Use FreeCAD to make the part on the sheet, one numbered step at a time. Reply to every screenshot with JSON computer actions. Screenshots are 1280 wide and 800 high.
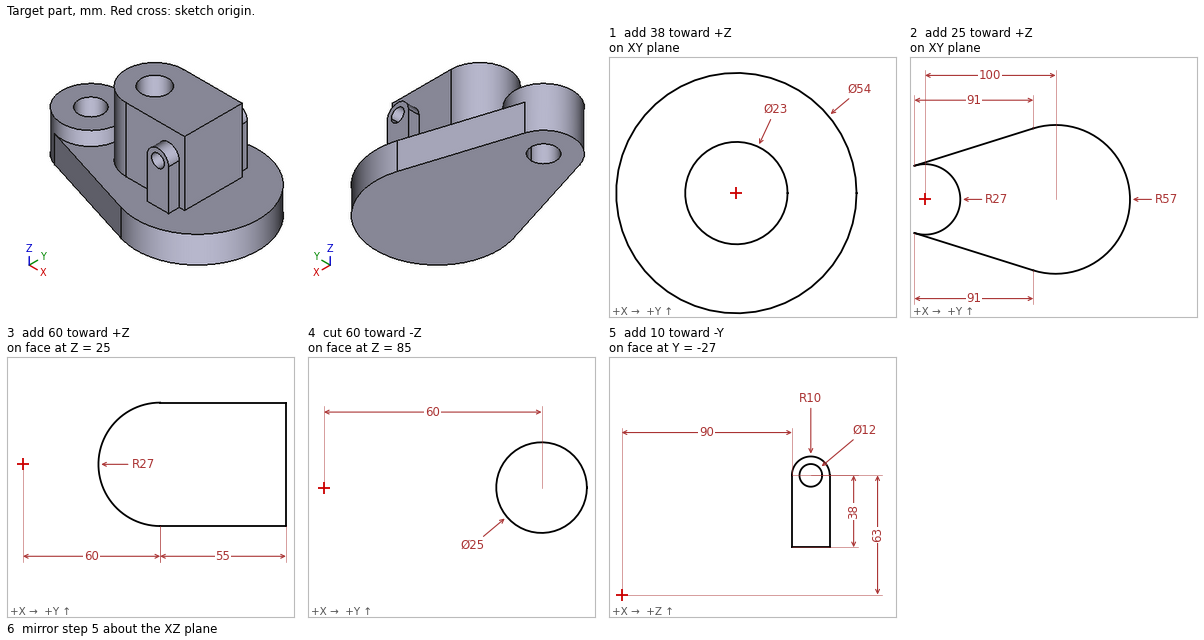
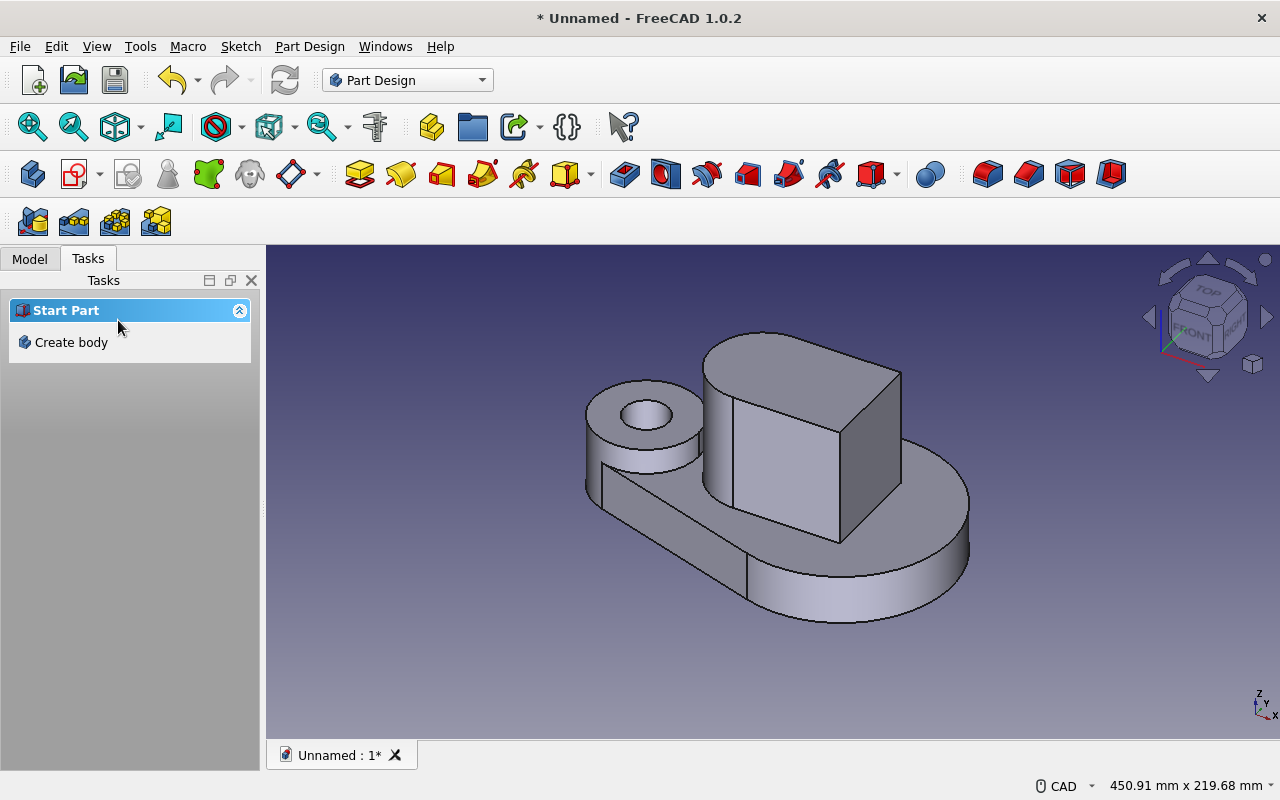
{"action": "left_click", "coordinate": [813, 383]}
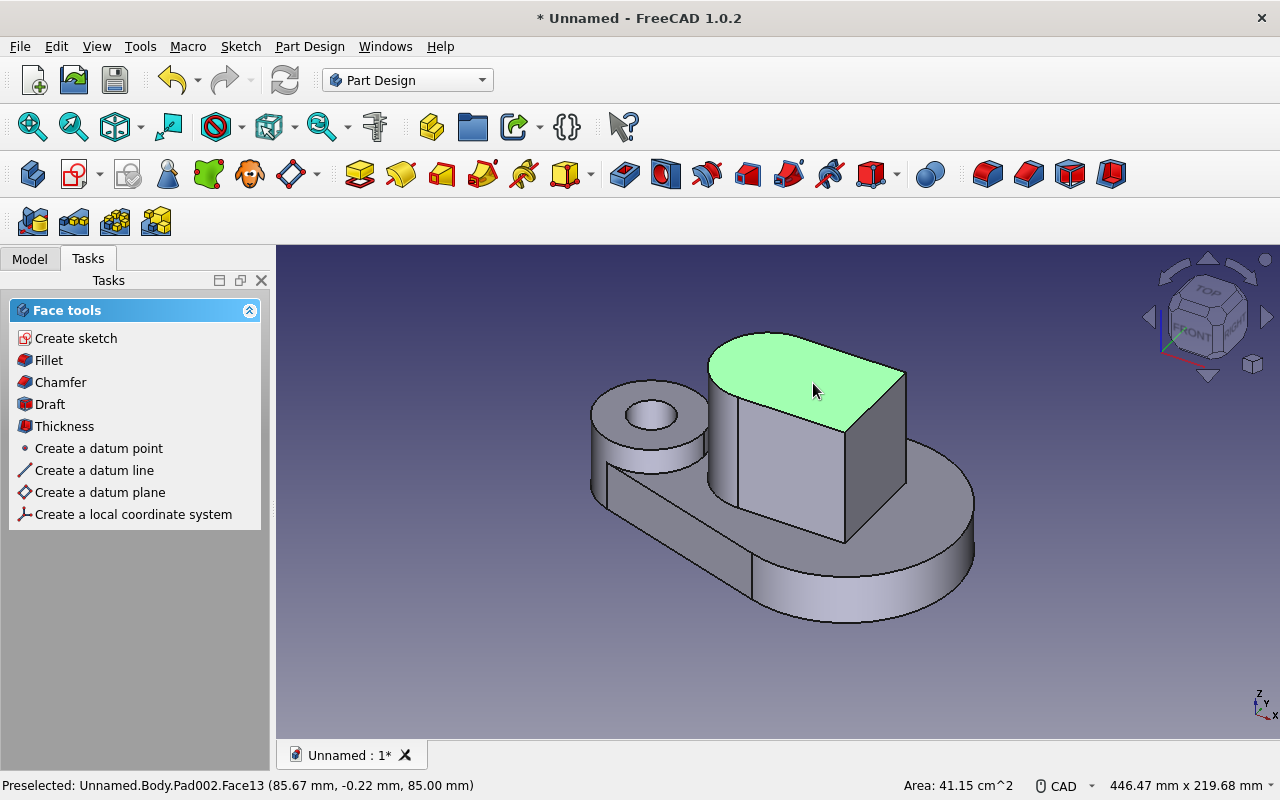
{"action": "left_click", "coordinate": [74, 174]}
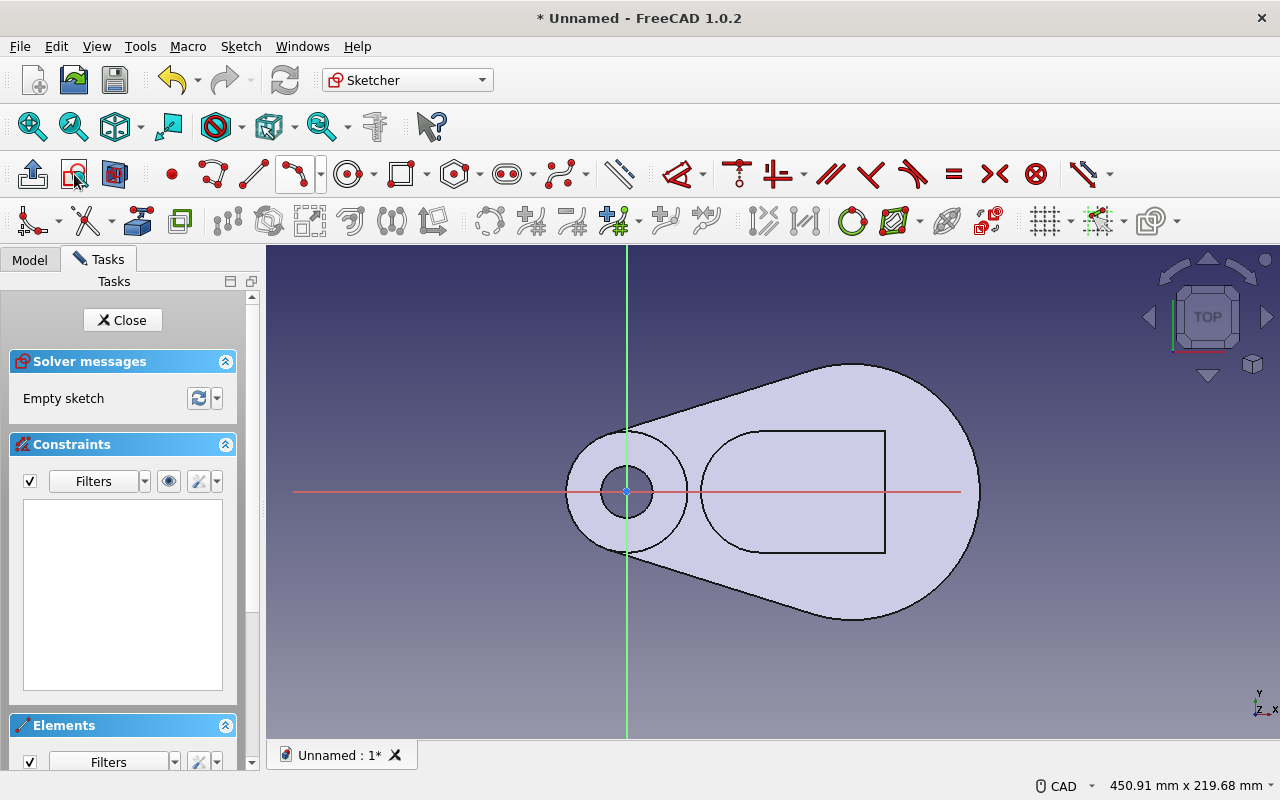
{"action": "scroll", "coordinate": [773, 492], "scroll_direction": "up", "scroll_amount": 9}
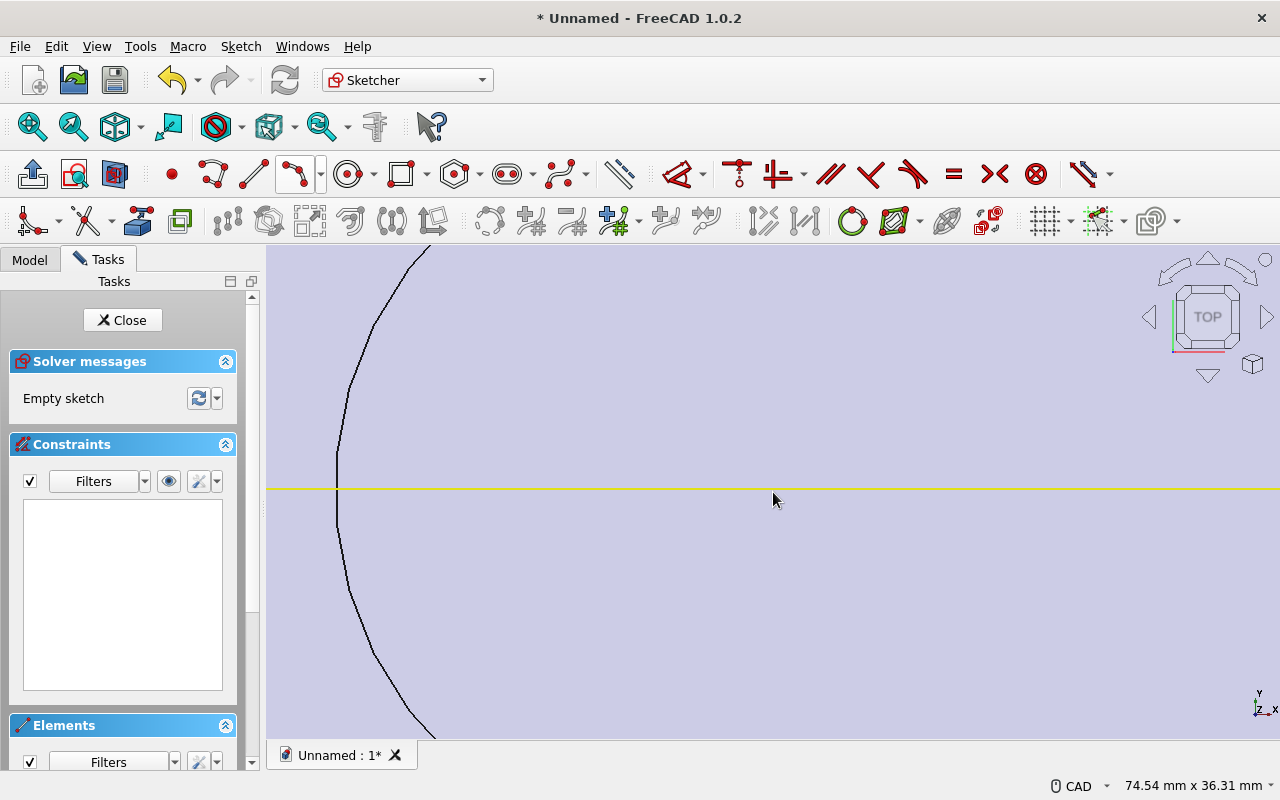
{"action": "key", "text": "g c"}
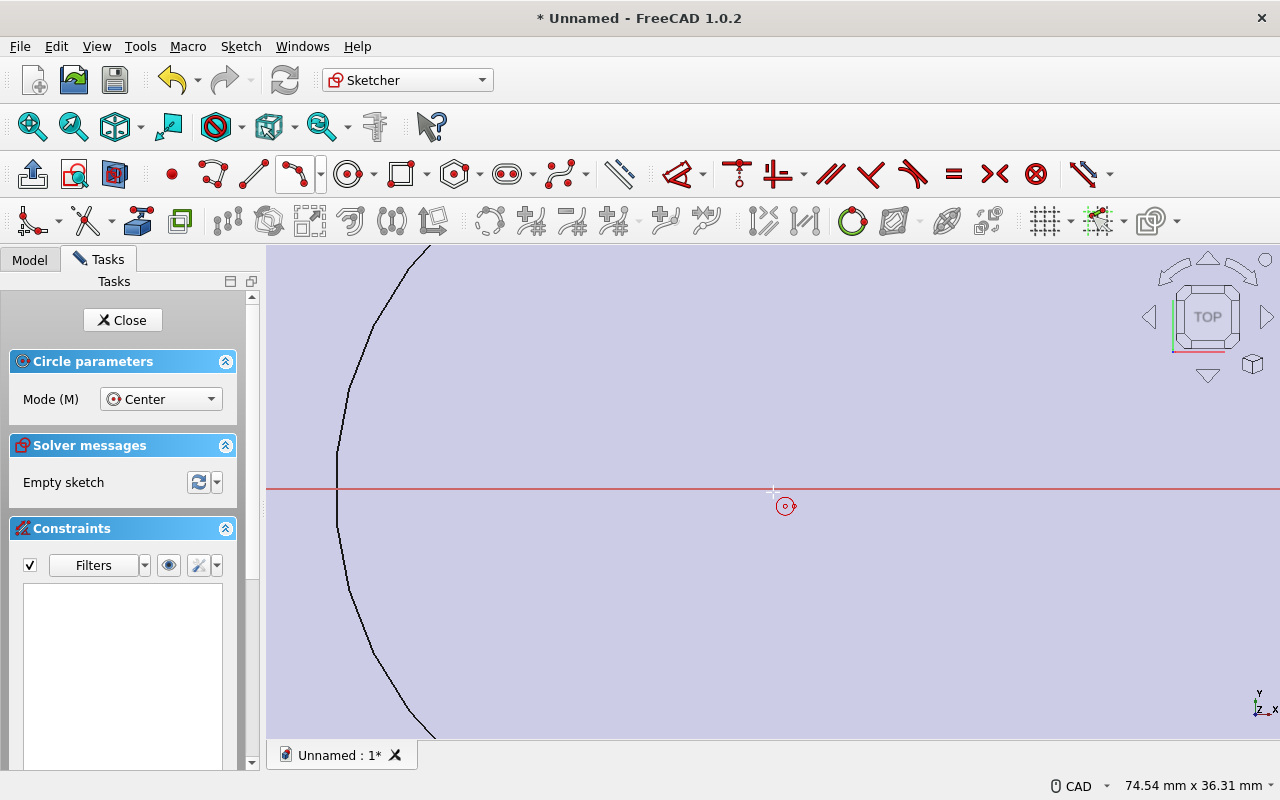
{"action": "left_click", "coordinate": [702, 489]}
{"action": "mouse_move", "coordinate": [823, 369]}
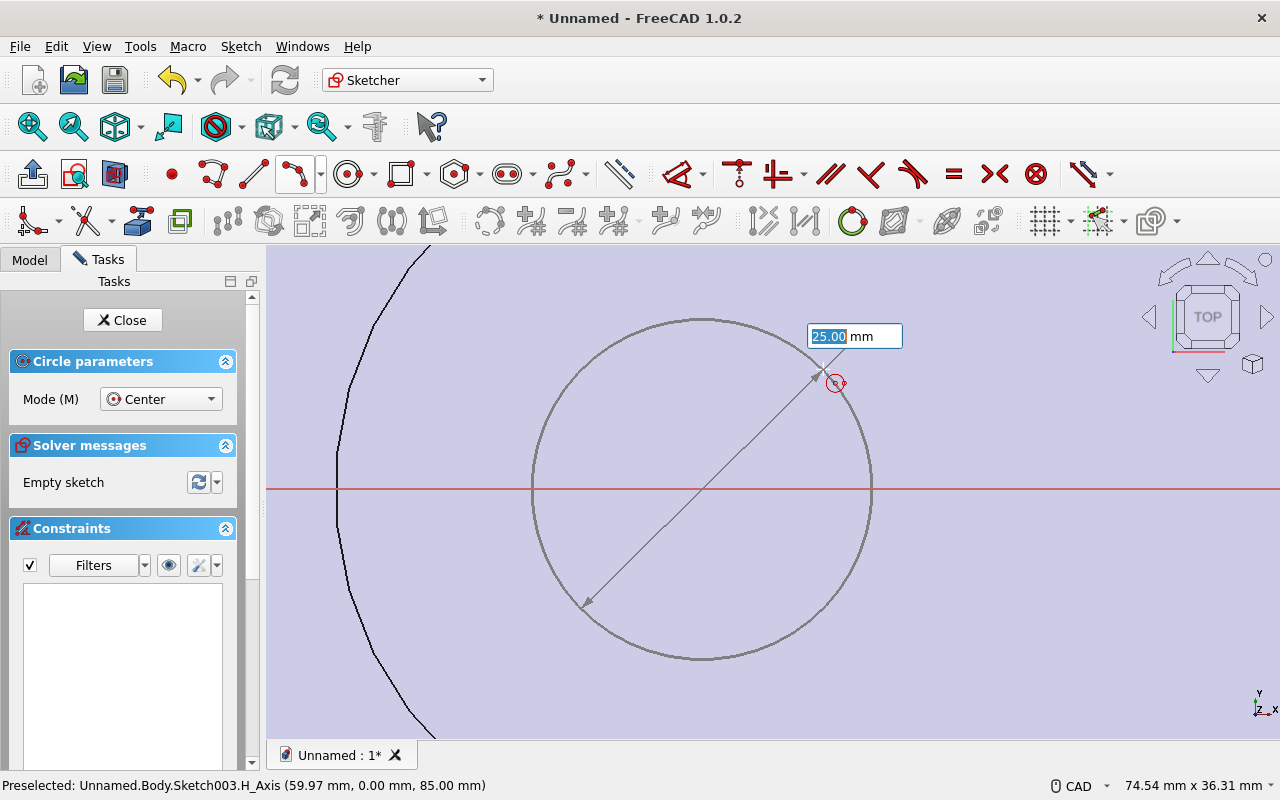
{"action": "type", "text": "25"}
{"action": "key", "text": "Return"}
{"action": "key", "text": "Escape"}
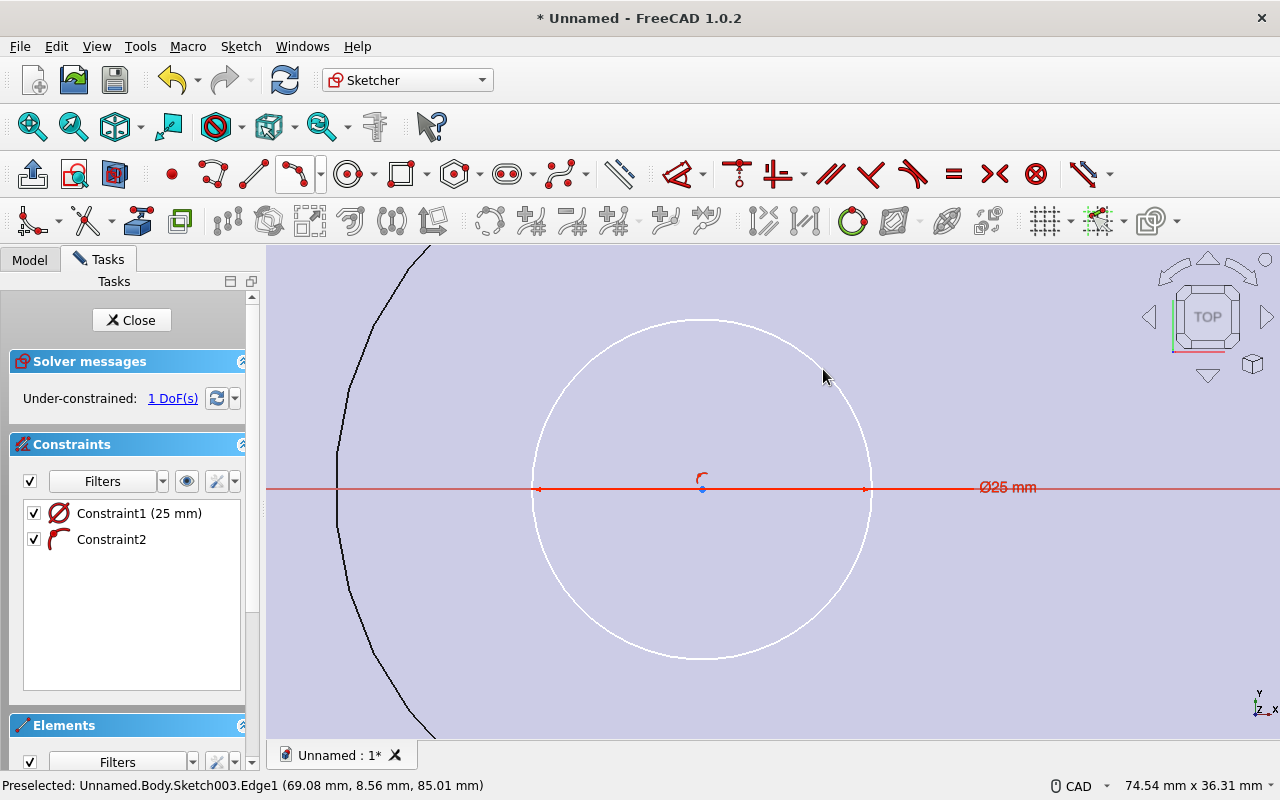
{"action": "key", "text": "d"}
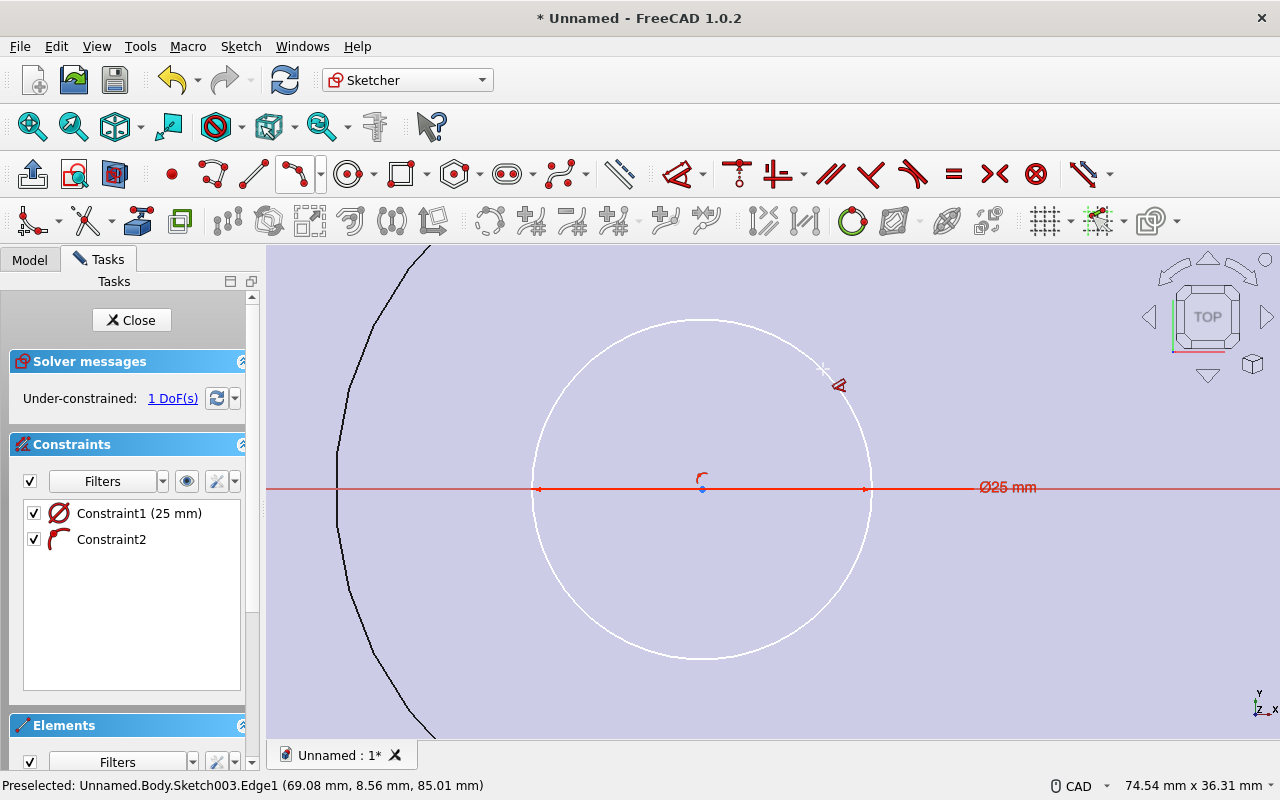
{"action": "left_click", "coordinate": [702, 489]}
{"action": "left_click", "coordinate": [498, 523]}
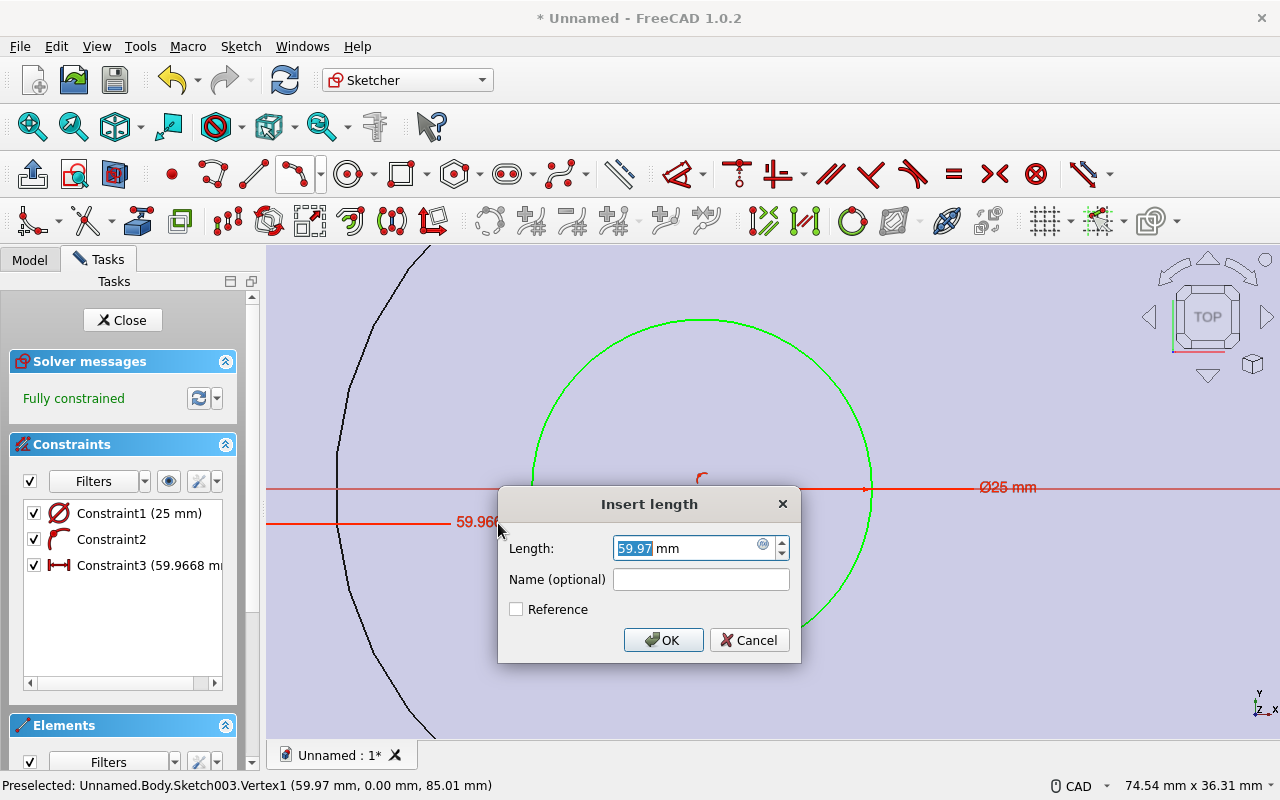
{"action": "type", "text": "60"}
{"action": "key", "text": "Return"}
{"action": "key", "text": "Escape"}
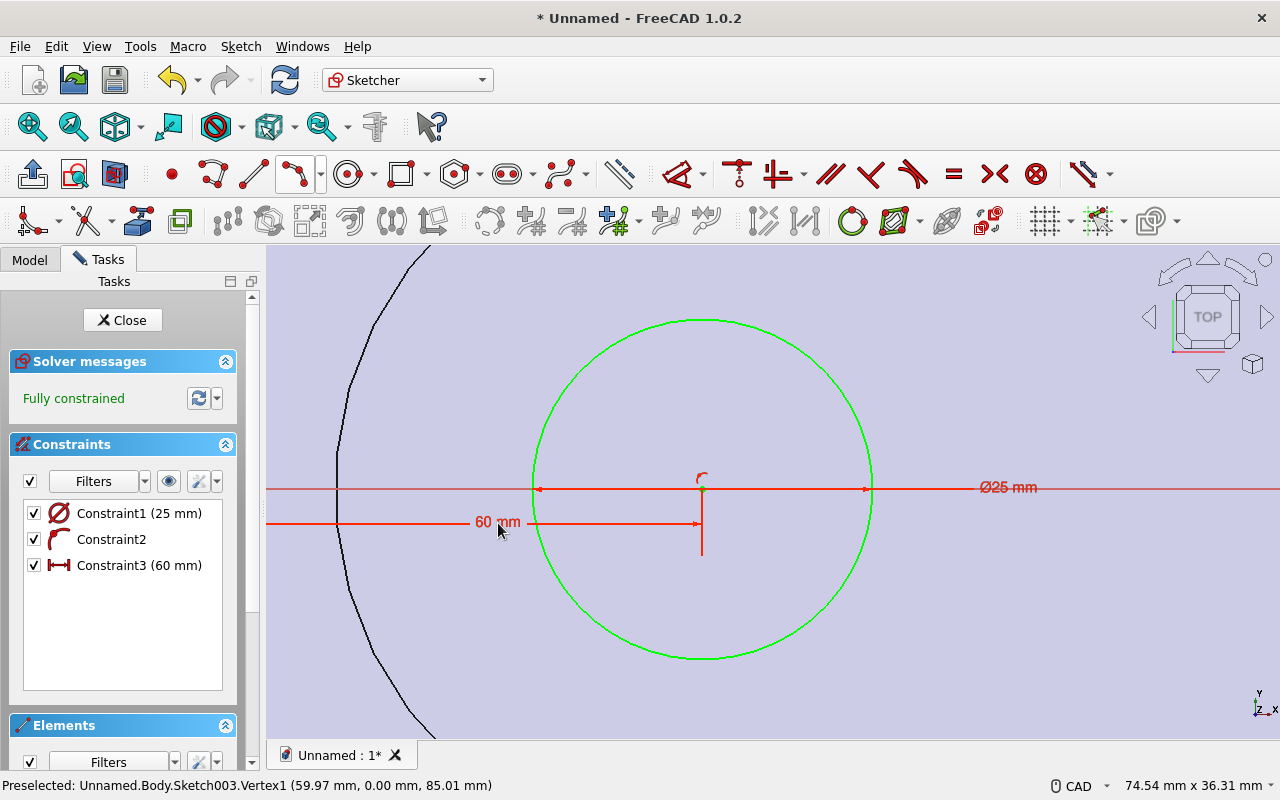
{"action": "left_click", "coordinate": [123, 320]}